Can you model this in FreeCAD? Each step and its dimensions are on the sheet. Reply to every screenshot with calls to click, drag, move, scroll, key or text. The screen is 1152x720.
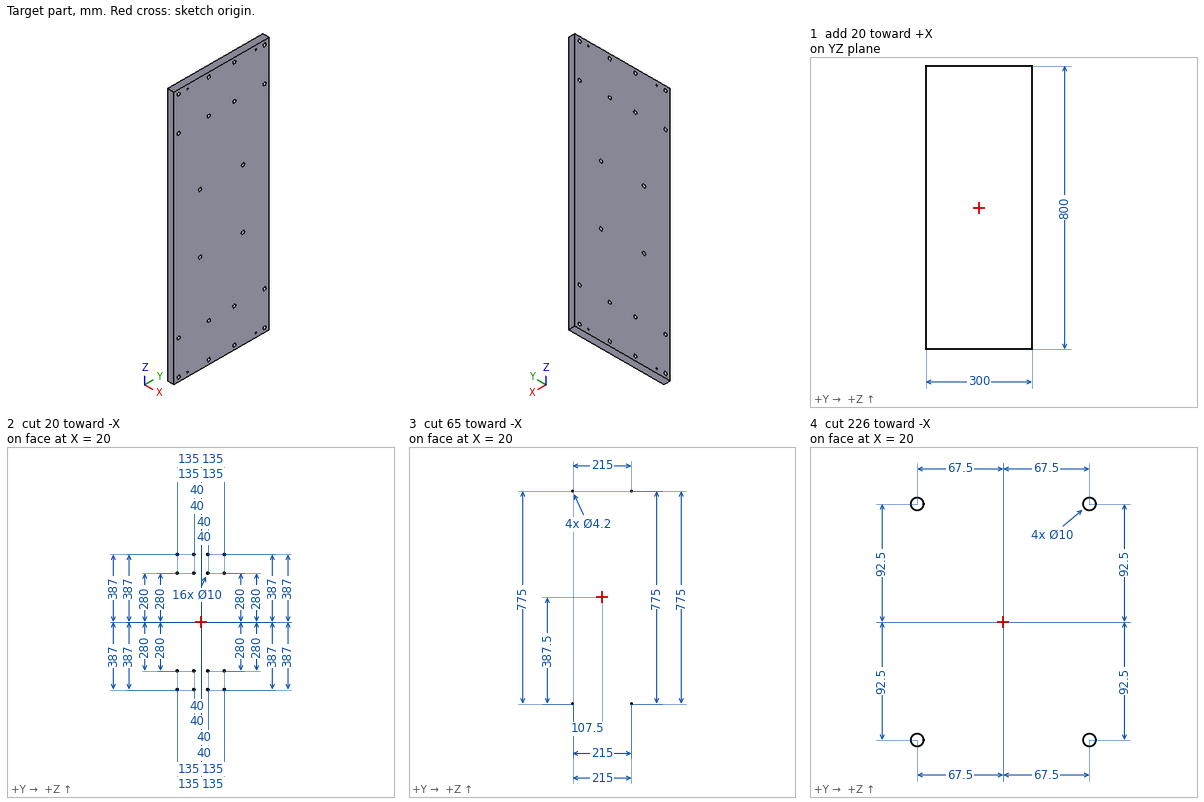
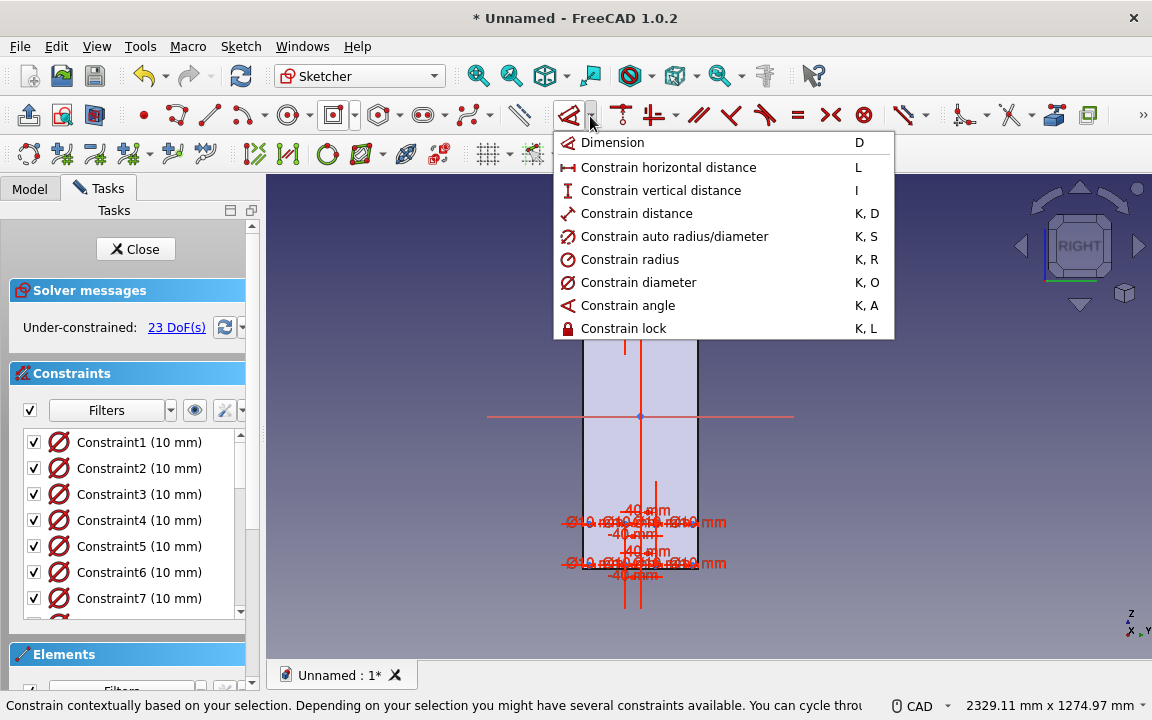
click(724, 190)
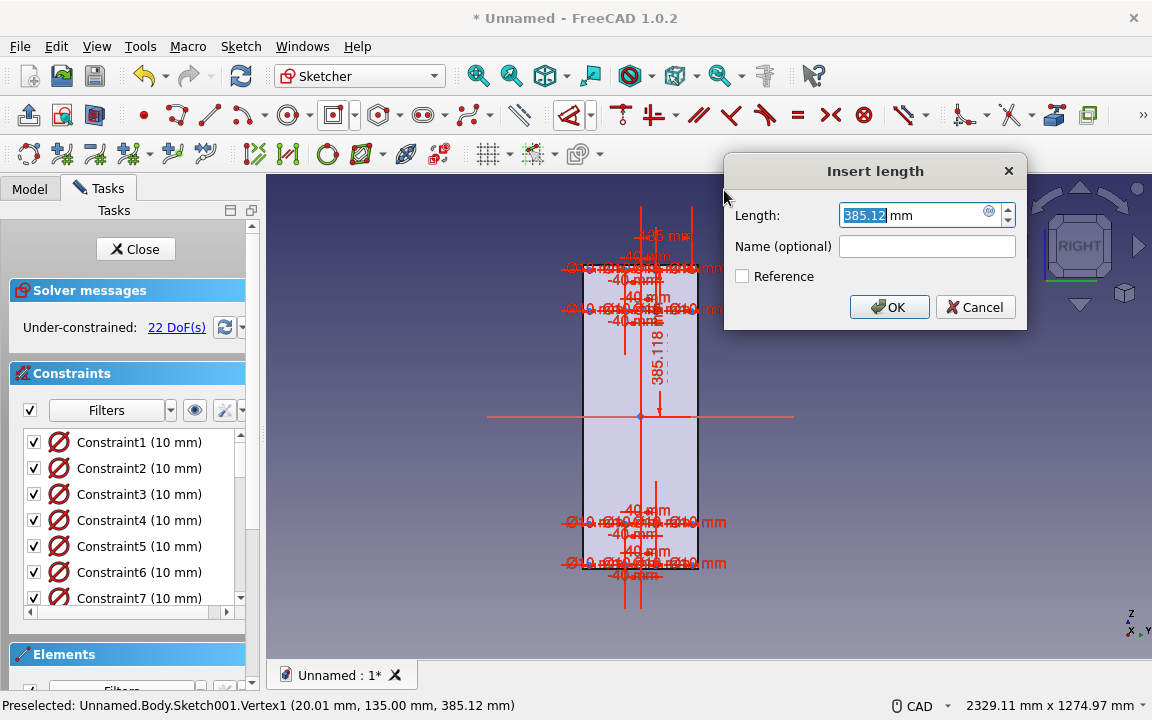
text(387)
key(Return)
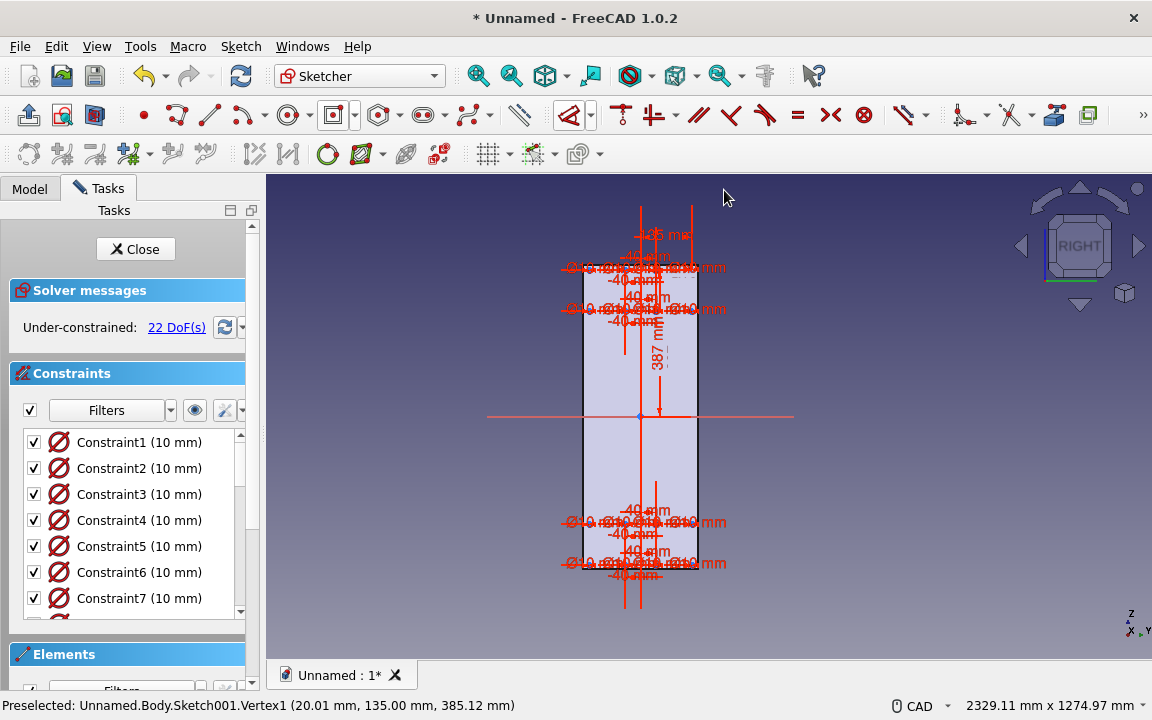
click(692, 311)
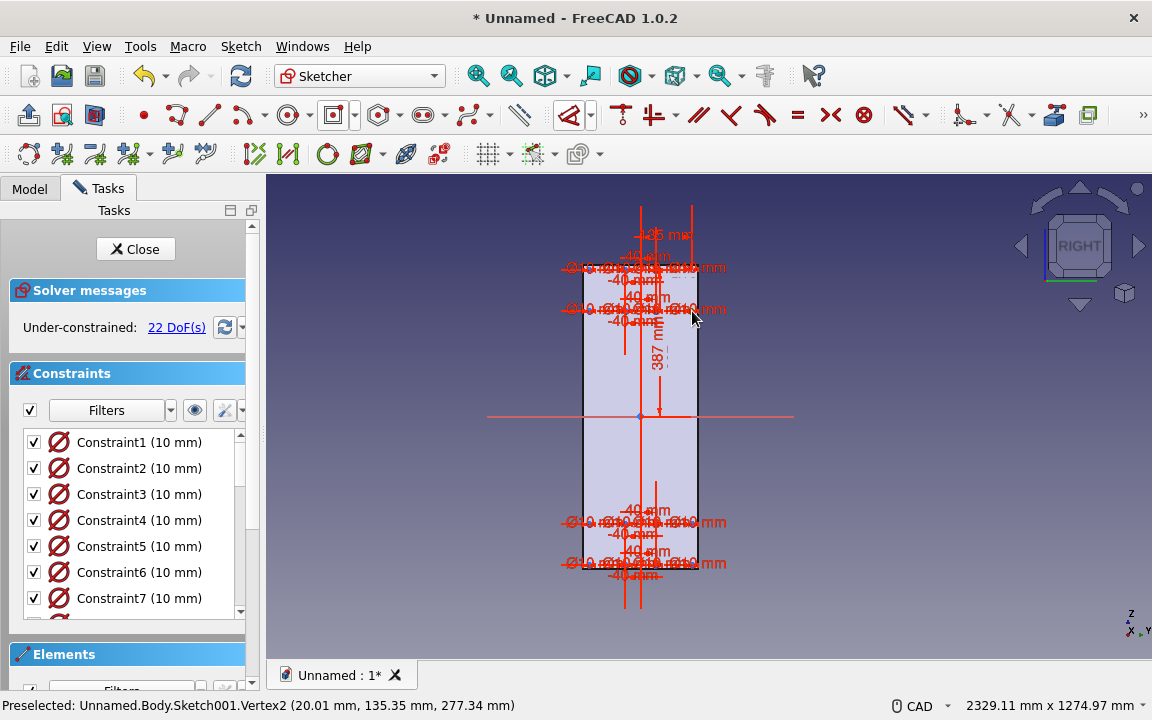
key(l)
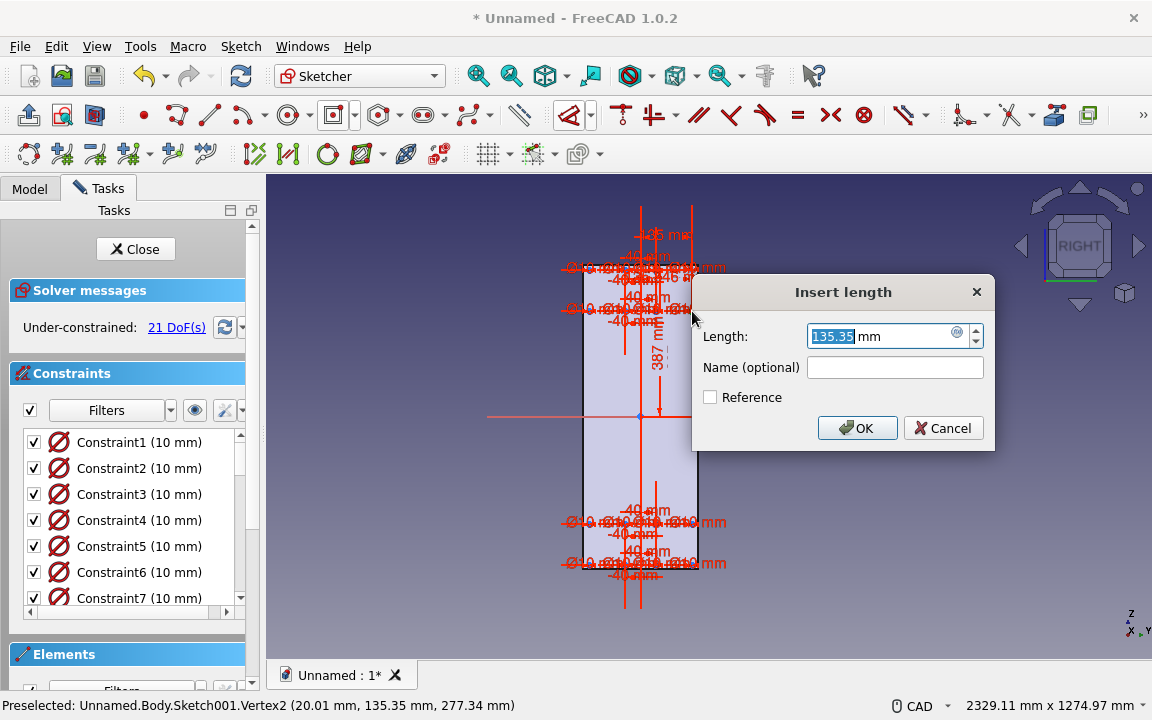
text(135)
key(Return)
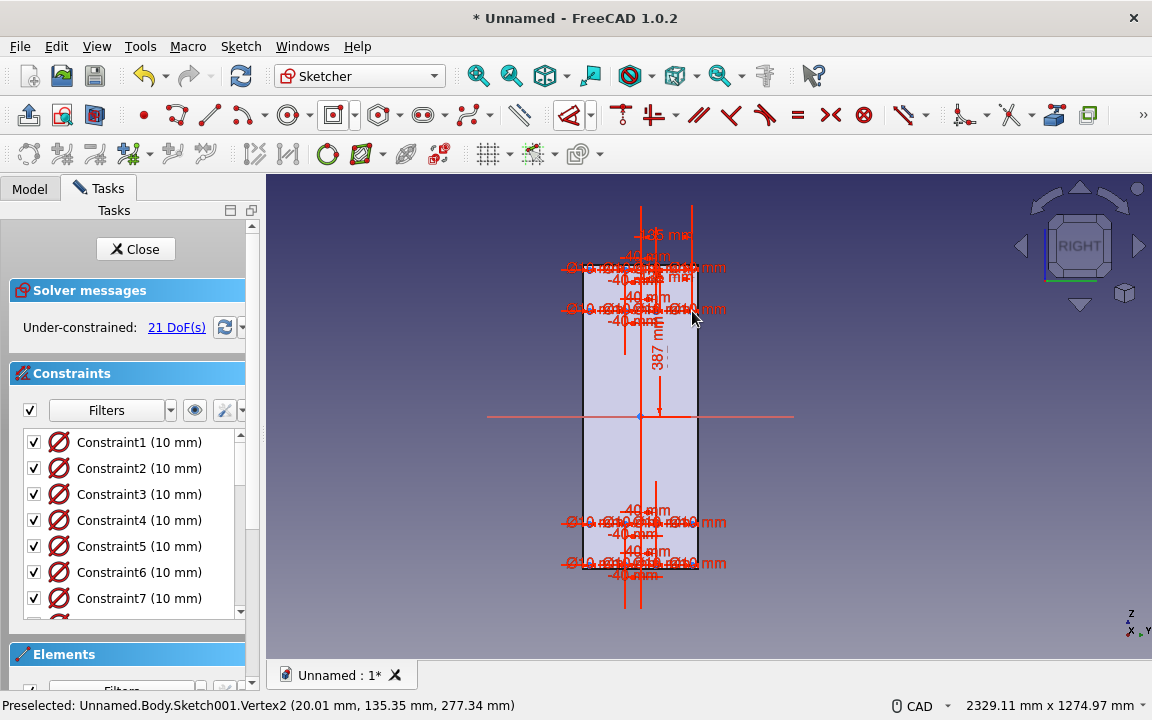
click(692, 311)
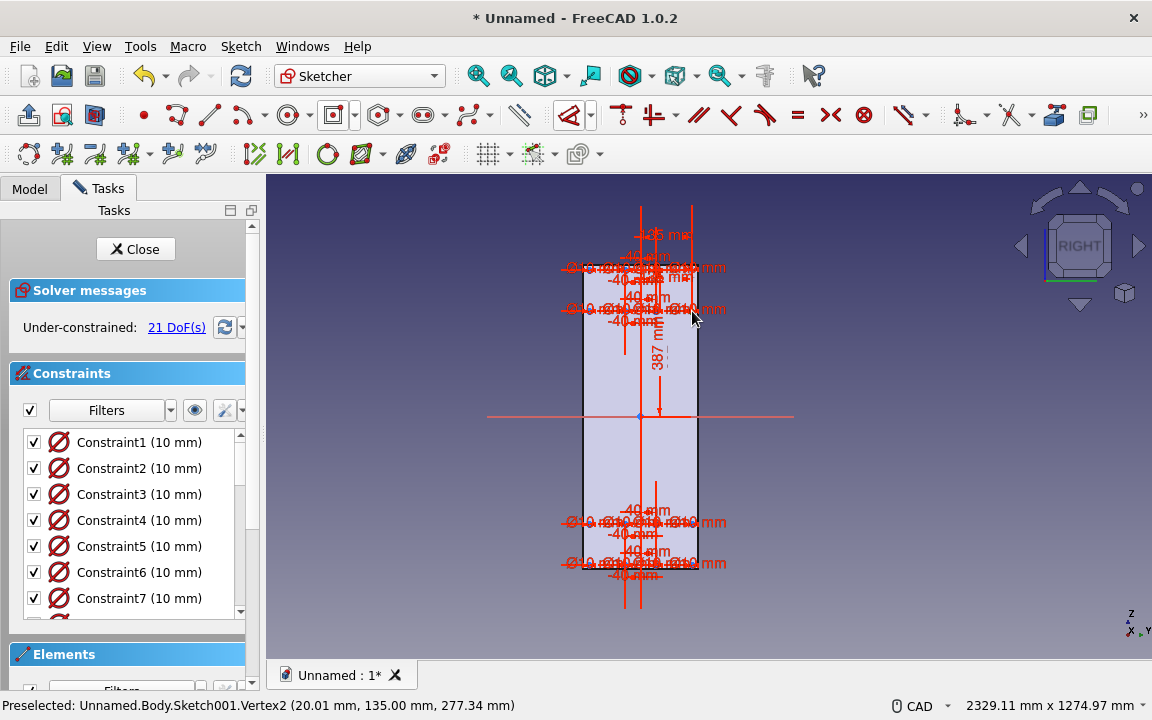
key(i)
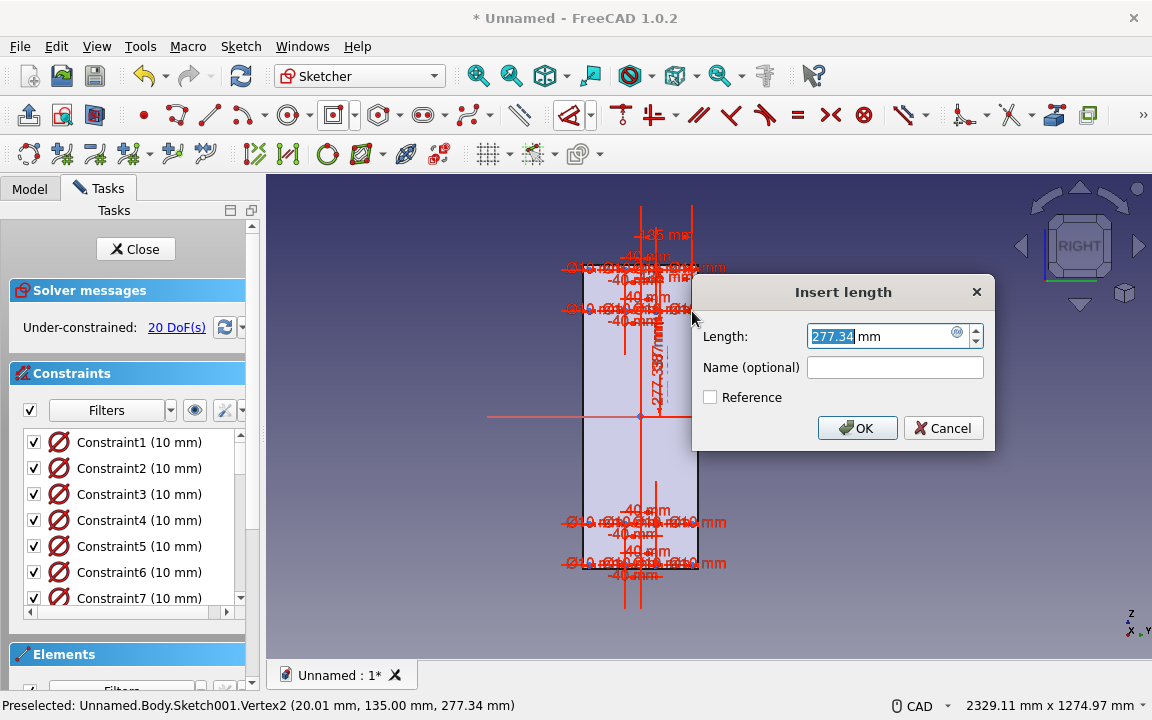
text(280)
key(Return)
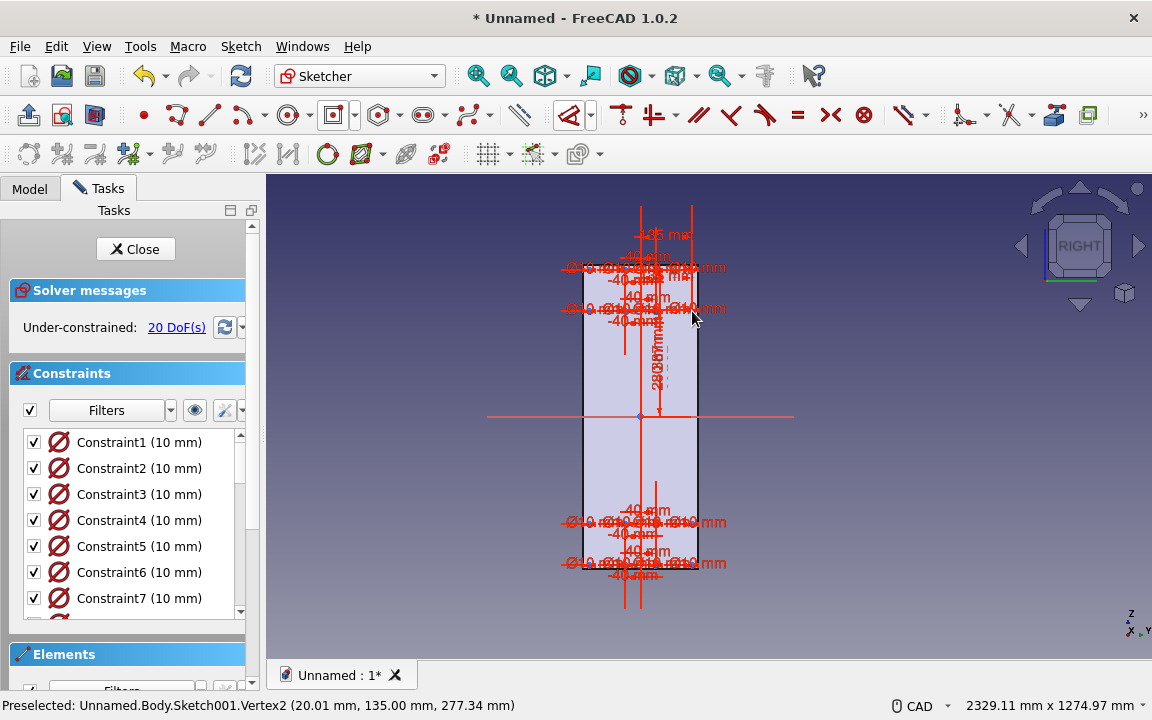
click(656, 311)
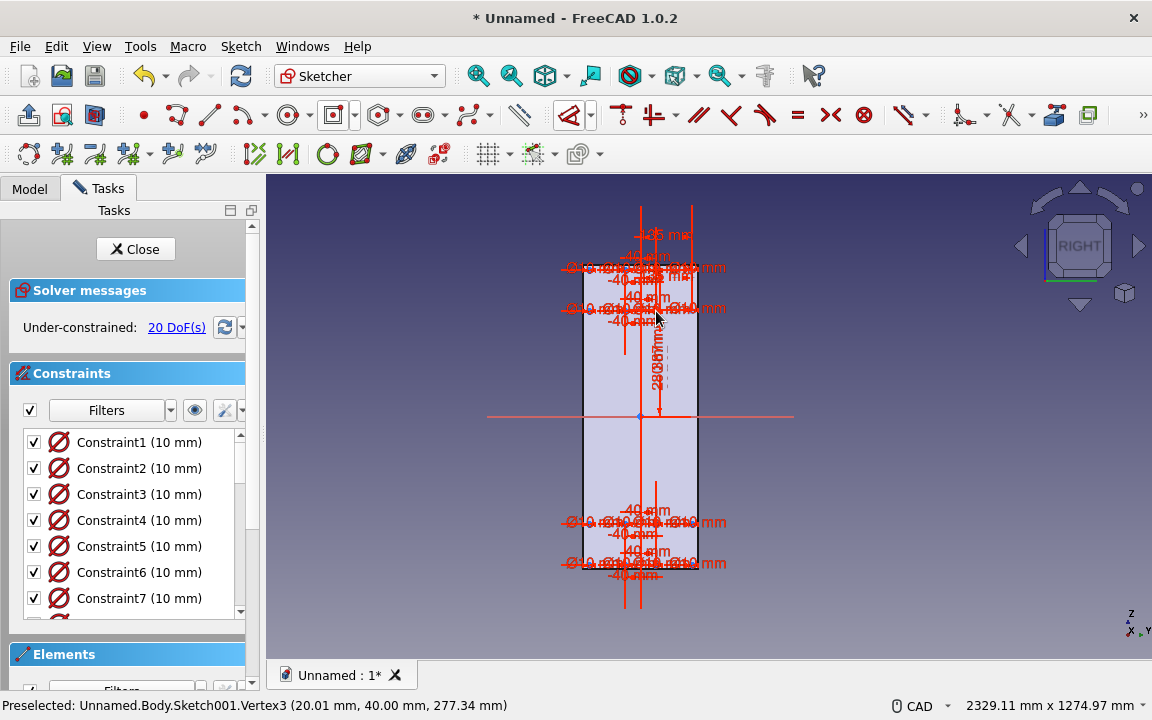
key(i)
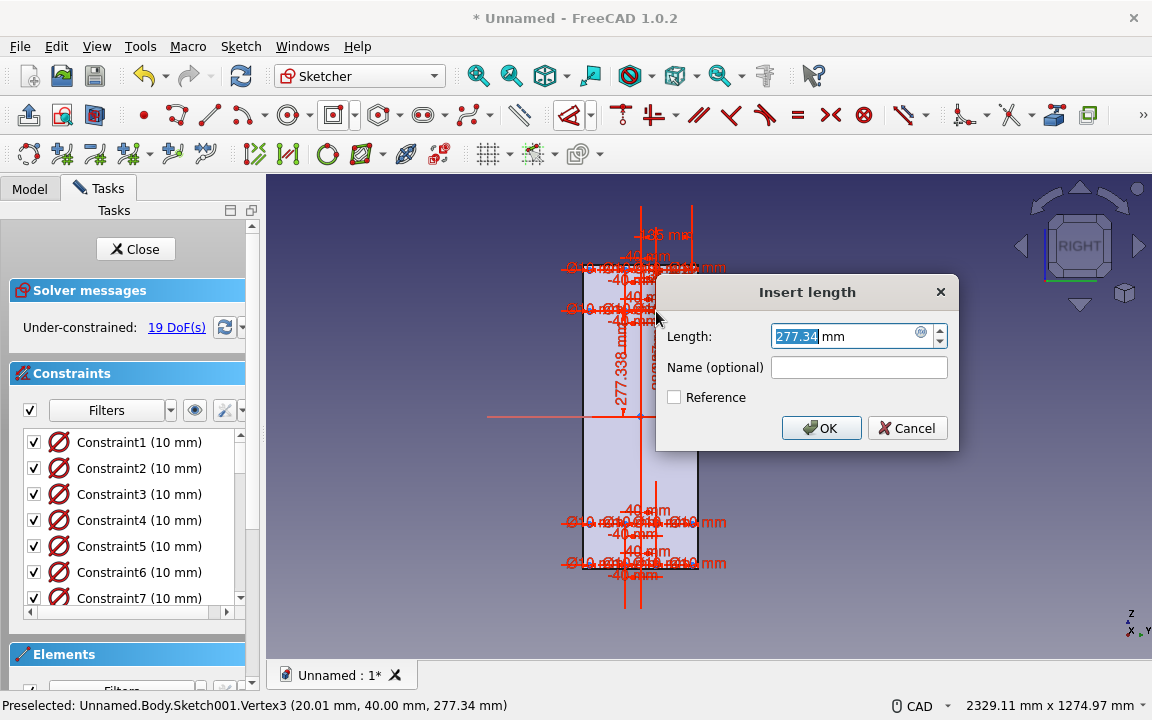
text(280)
key(Return)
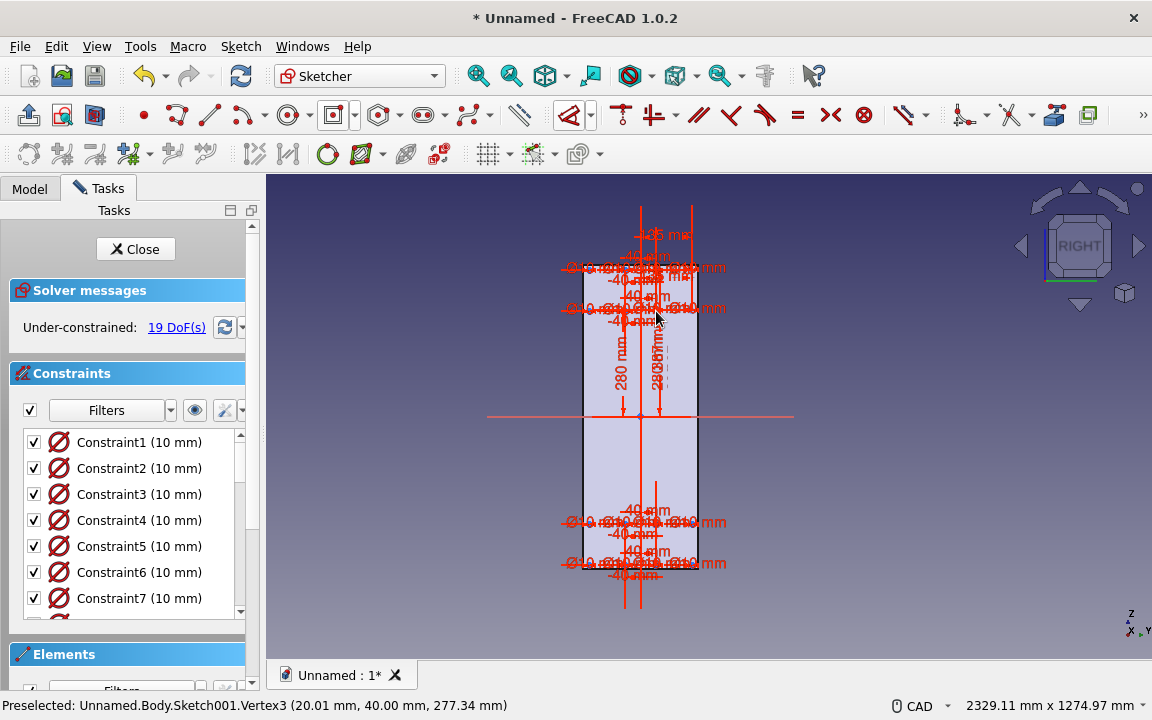
click(656, 270)